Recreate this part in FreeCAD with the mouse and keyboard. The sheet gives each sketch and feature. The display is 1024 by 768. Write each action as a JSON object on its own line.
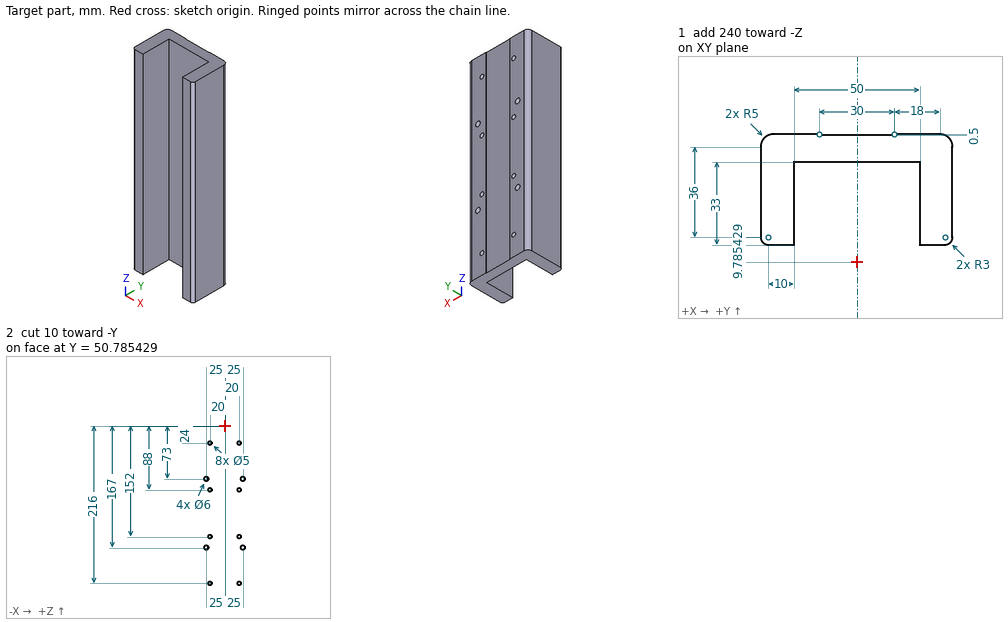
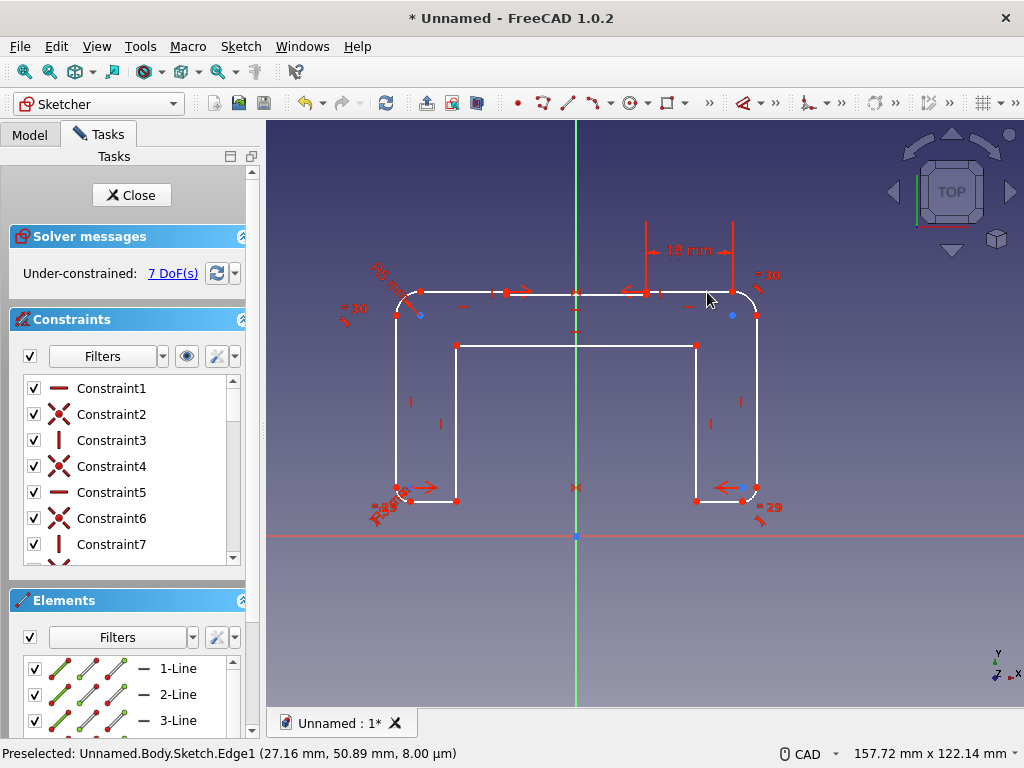
{"action": "left_click", "coordinate": [604, 295]}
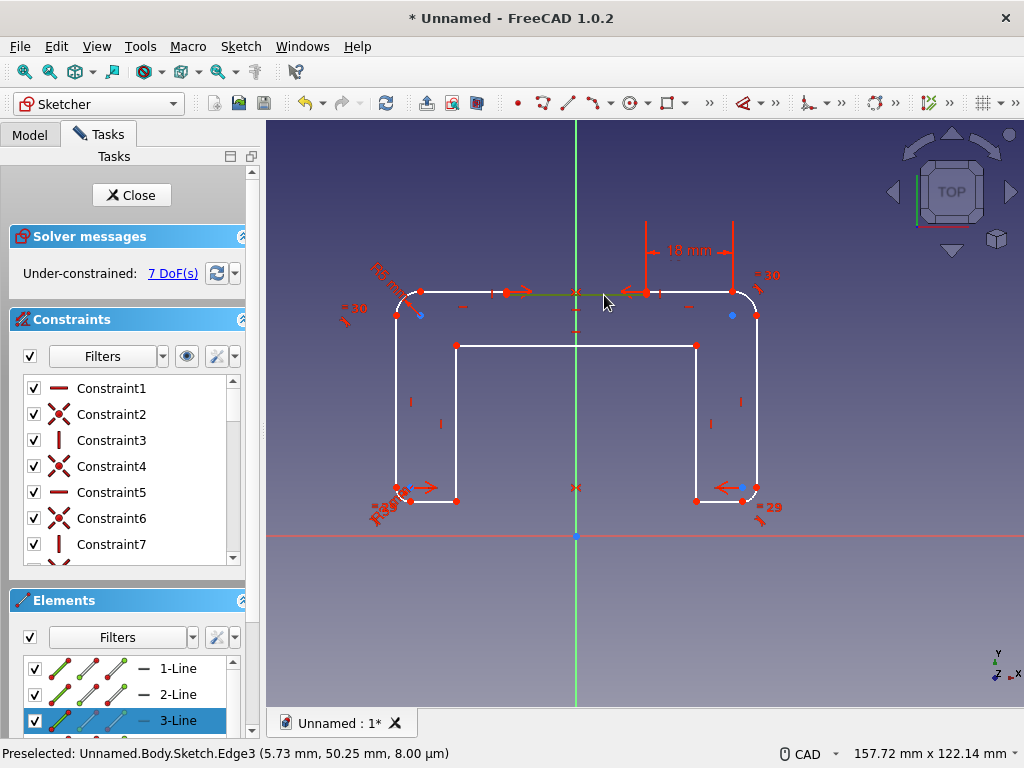
{"action": "key", "text": "l"}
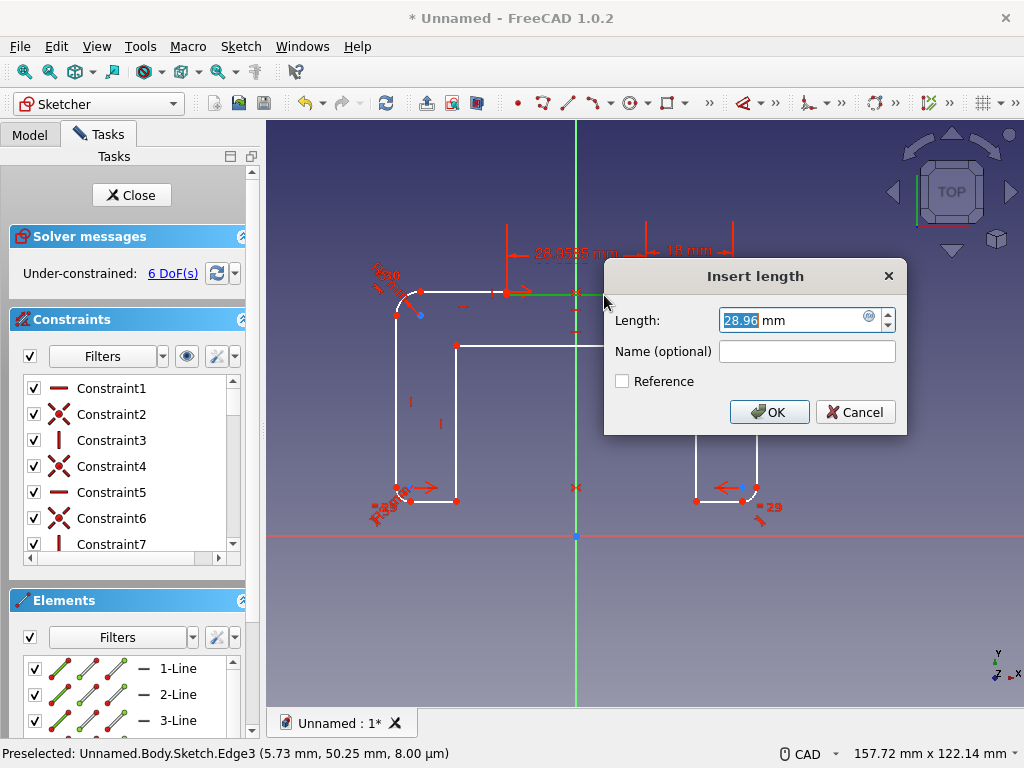
{"action": "type", "text": "30"}
{"action": "key", "text": "Return"}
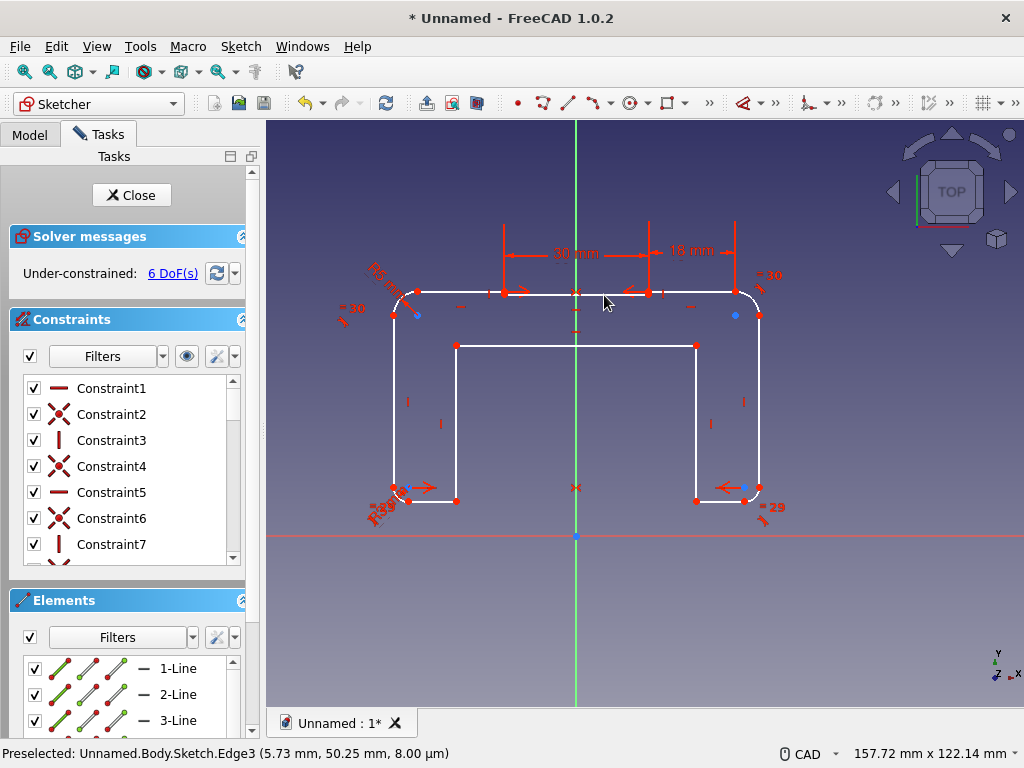
{"action": "left_click", "coordinate": [394, 367]}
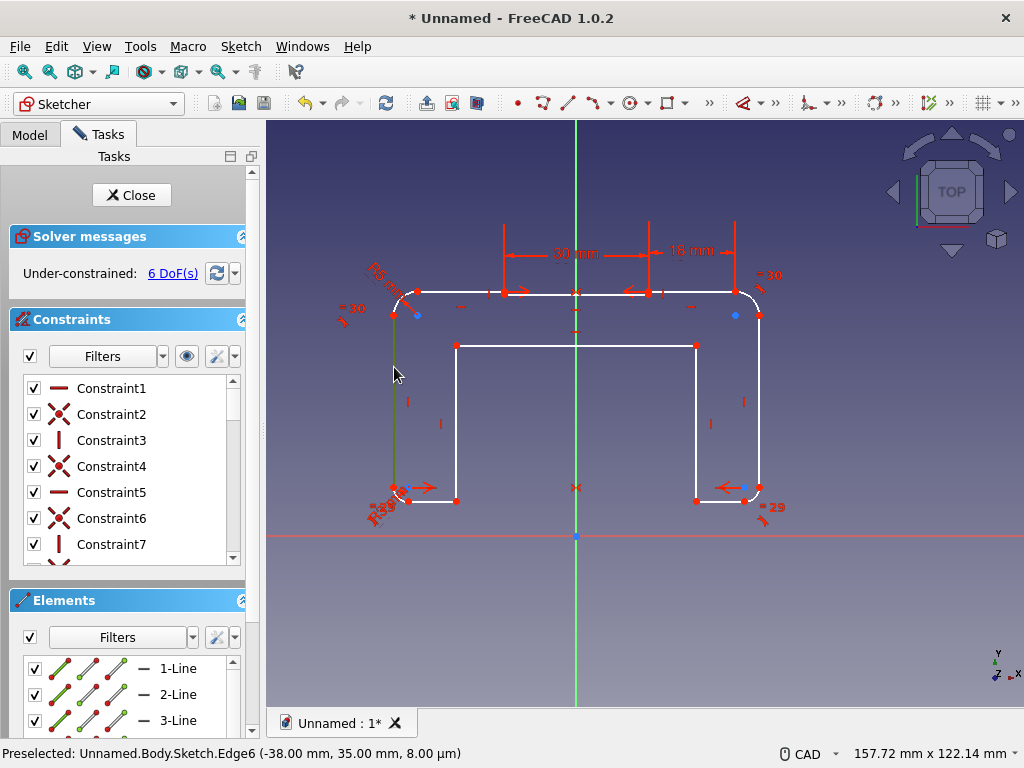
{"action": "key", "text": "i"}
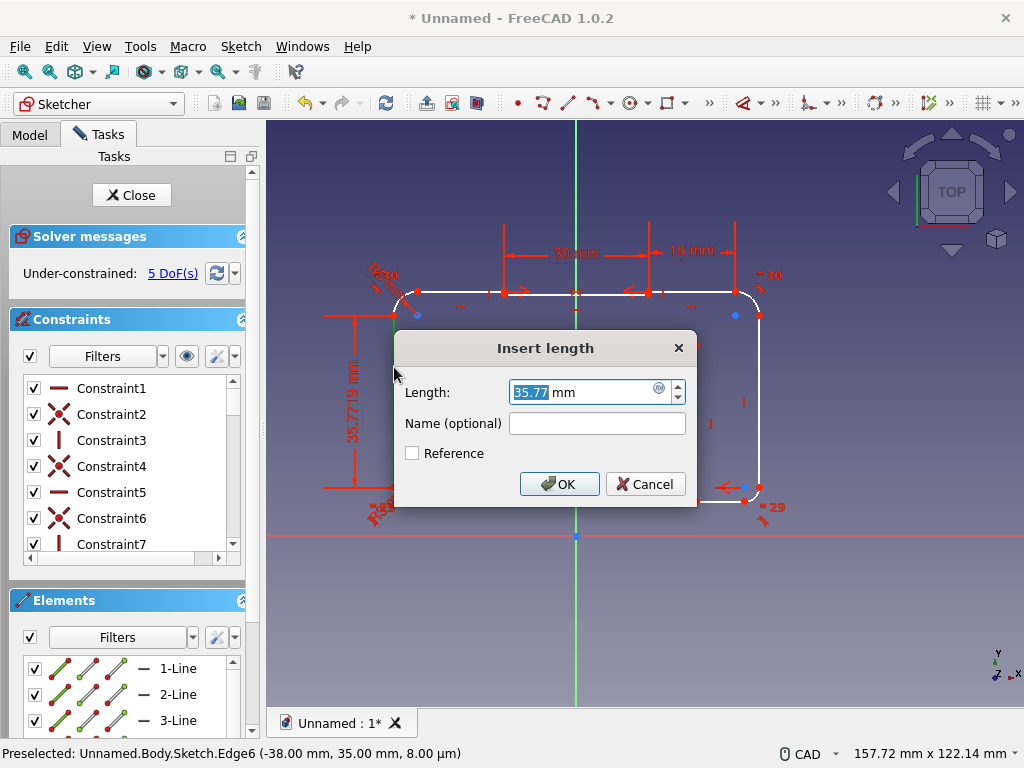
{"action": "type", "text": "36"}
{"action": "key", "text": "Return"}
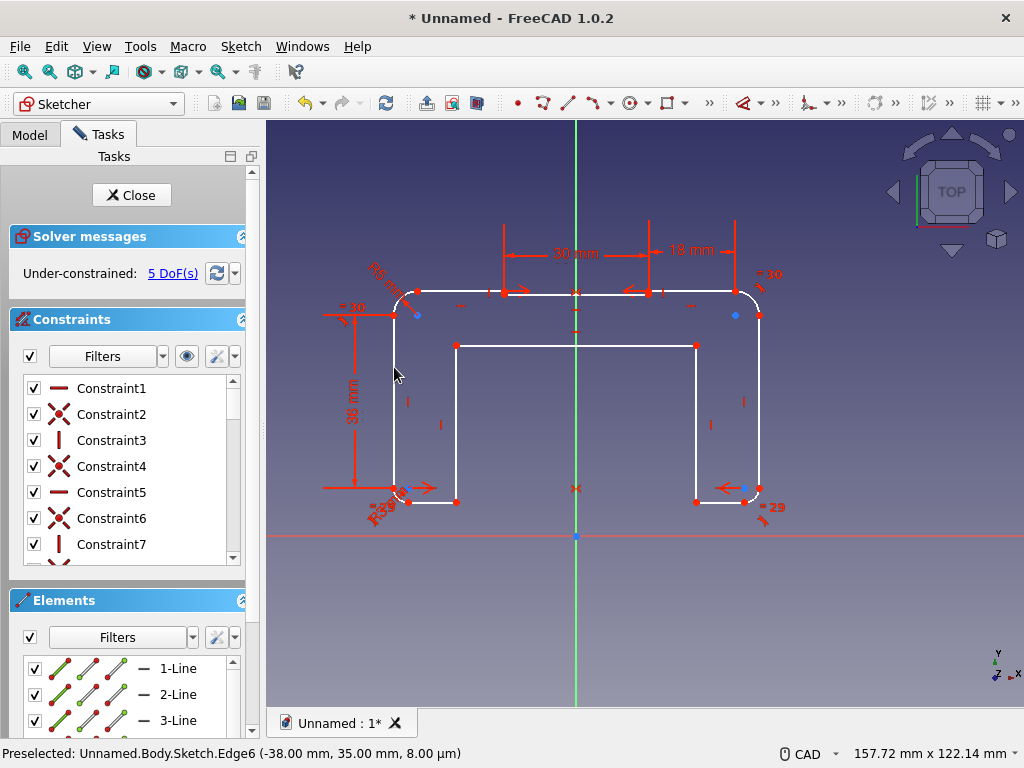
{"action": "left_click", "coordinate": [423, 503]}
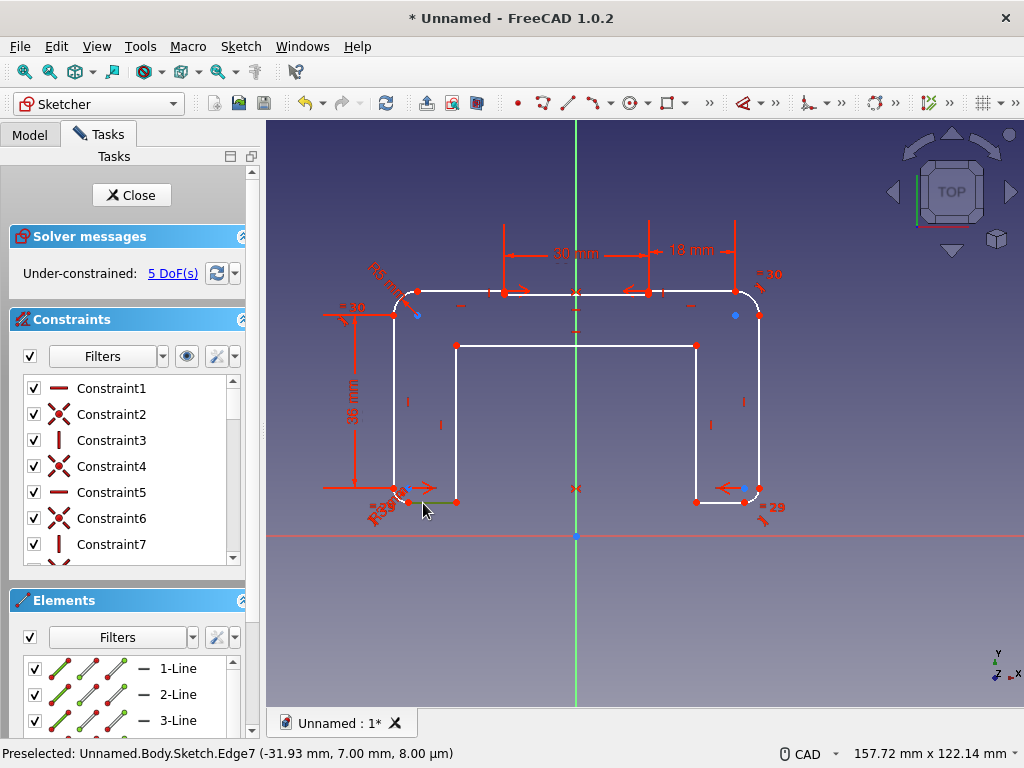
{"action": "key", "text": "l"}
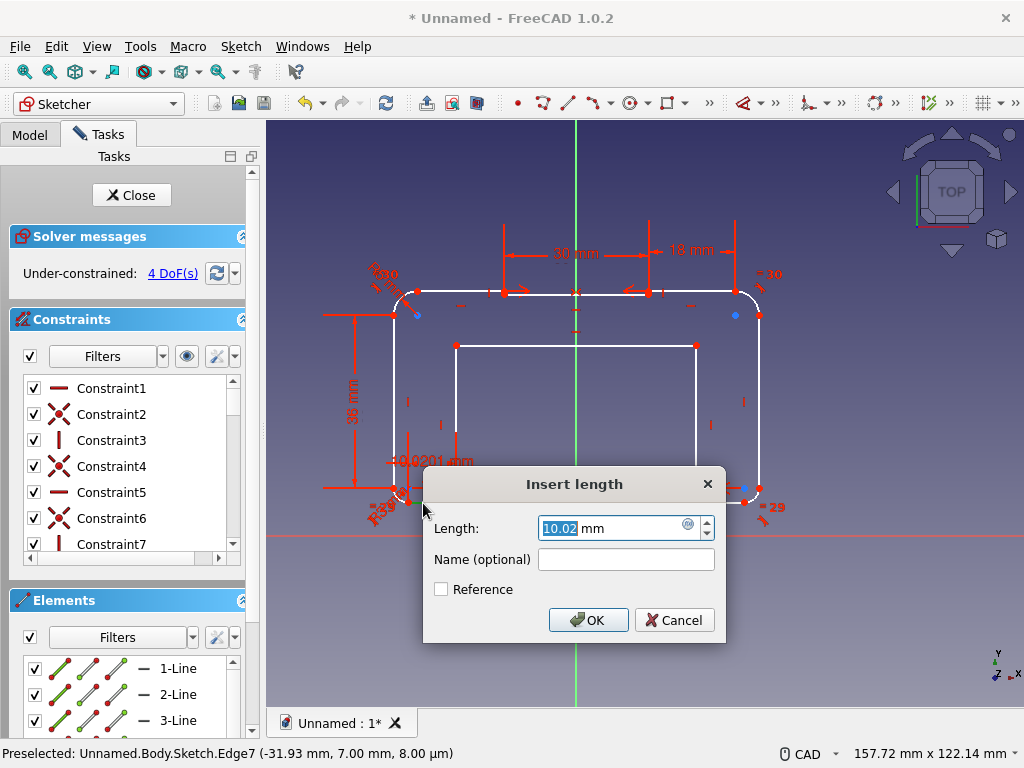
{"action": "type", "text": "10"}
{"action": "key", "text": "Return"}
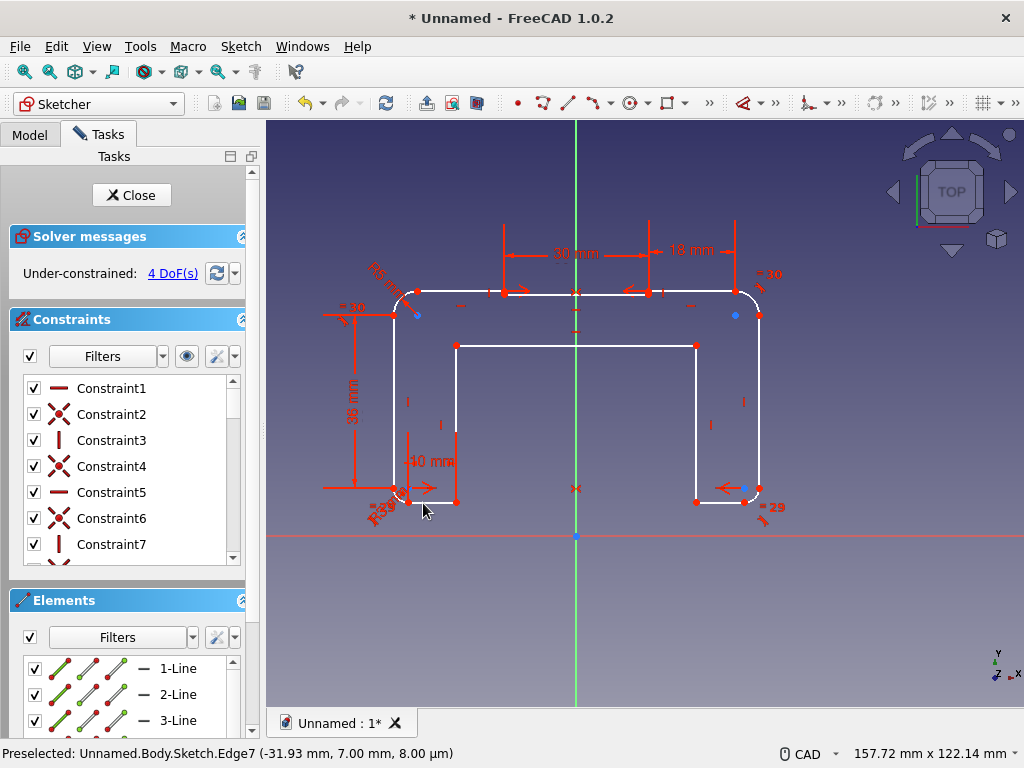
{"action": "left_click", "coordinate": [456, 456]}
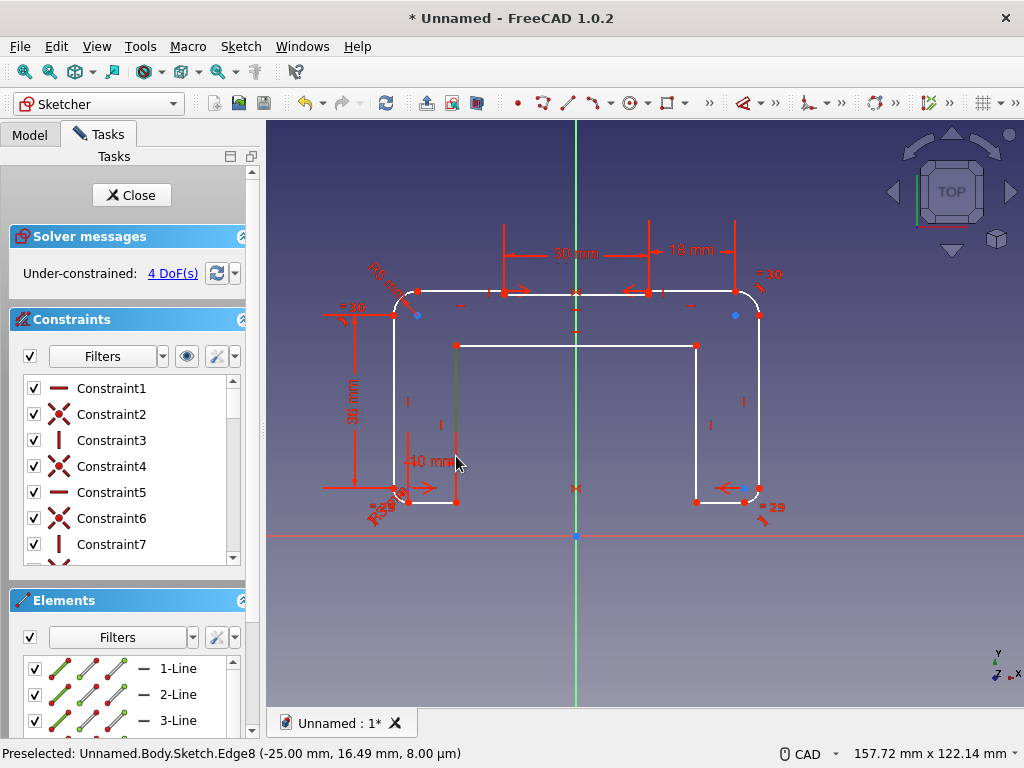
{"action": "key", "text": "i"}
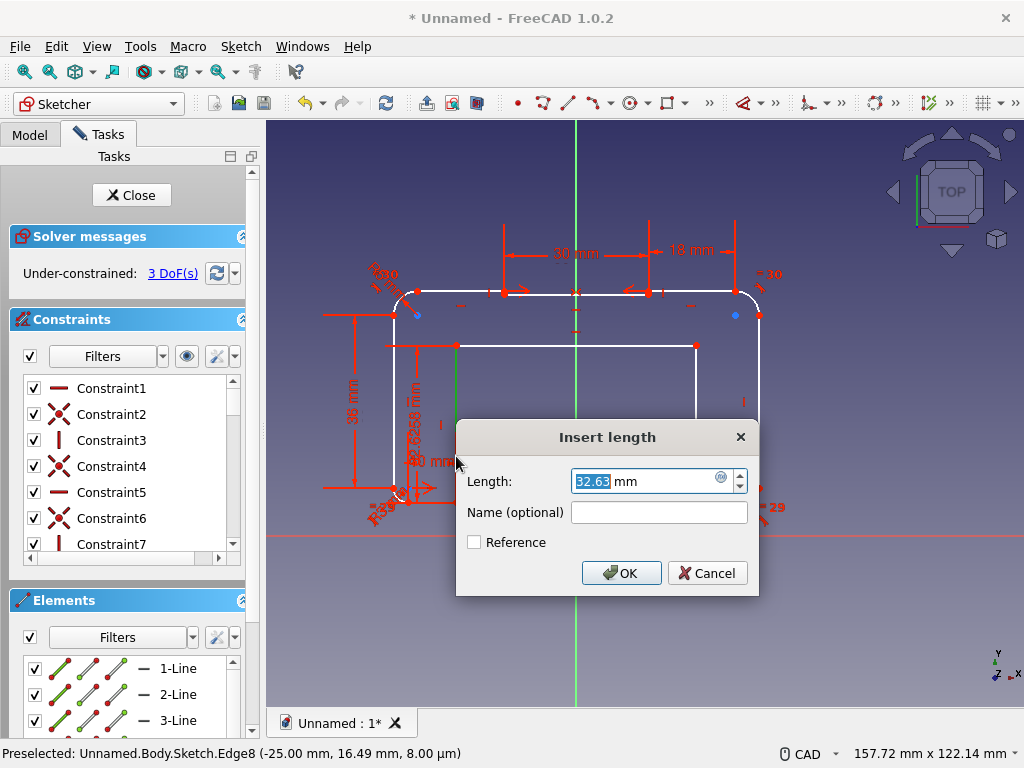
{"action": "type", "text": "33"}
{"action": "key", "text": "Return"}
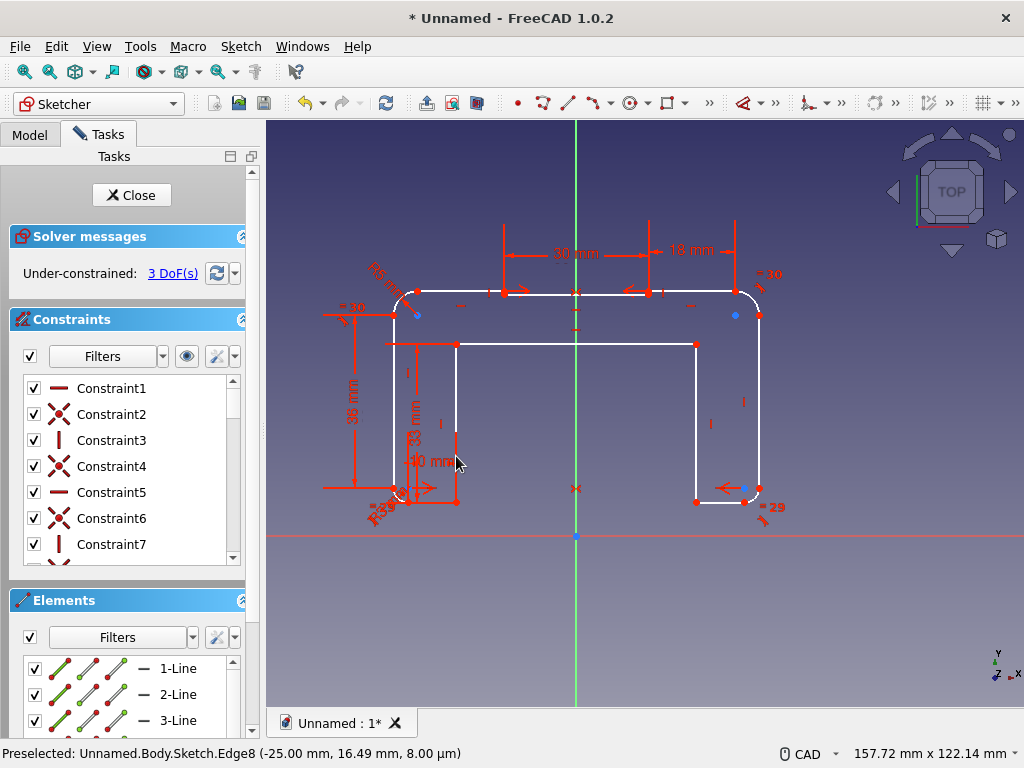
{"action": "left_click", "coordinate": [528, 344]}